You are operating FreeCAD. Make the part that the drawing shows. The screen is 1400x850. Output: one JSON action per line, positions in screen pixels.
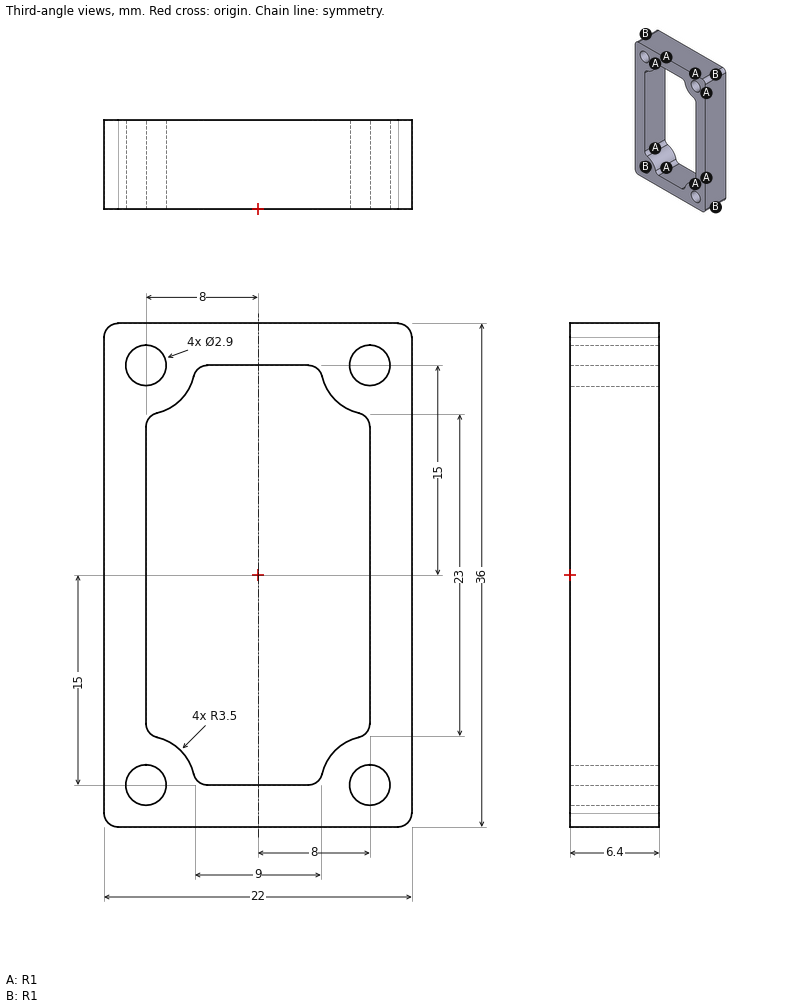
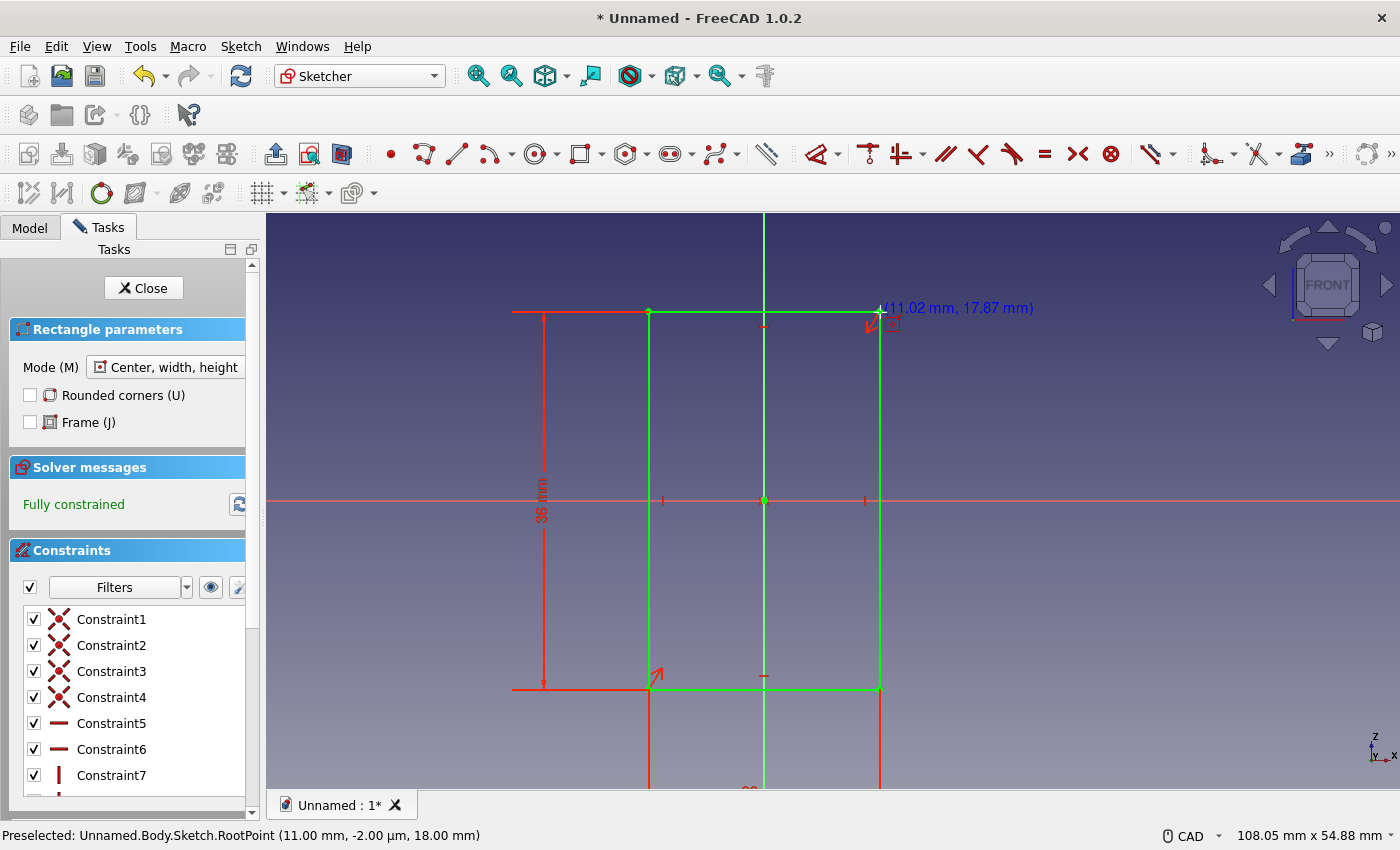
{"action": "left_click", "coordinate": [457, 154]}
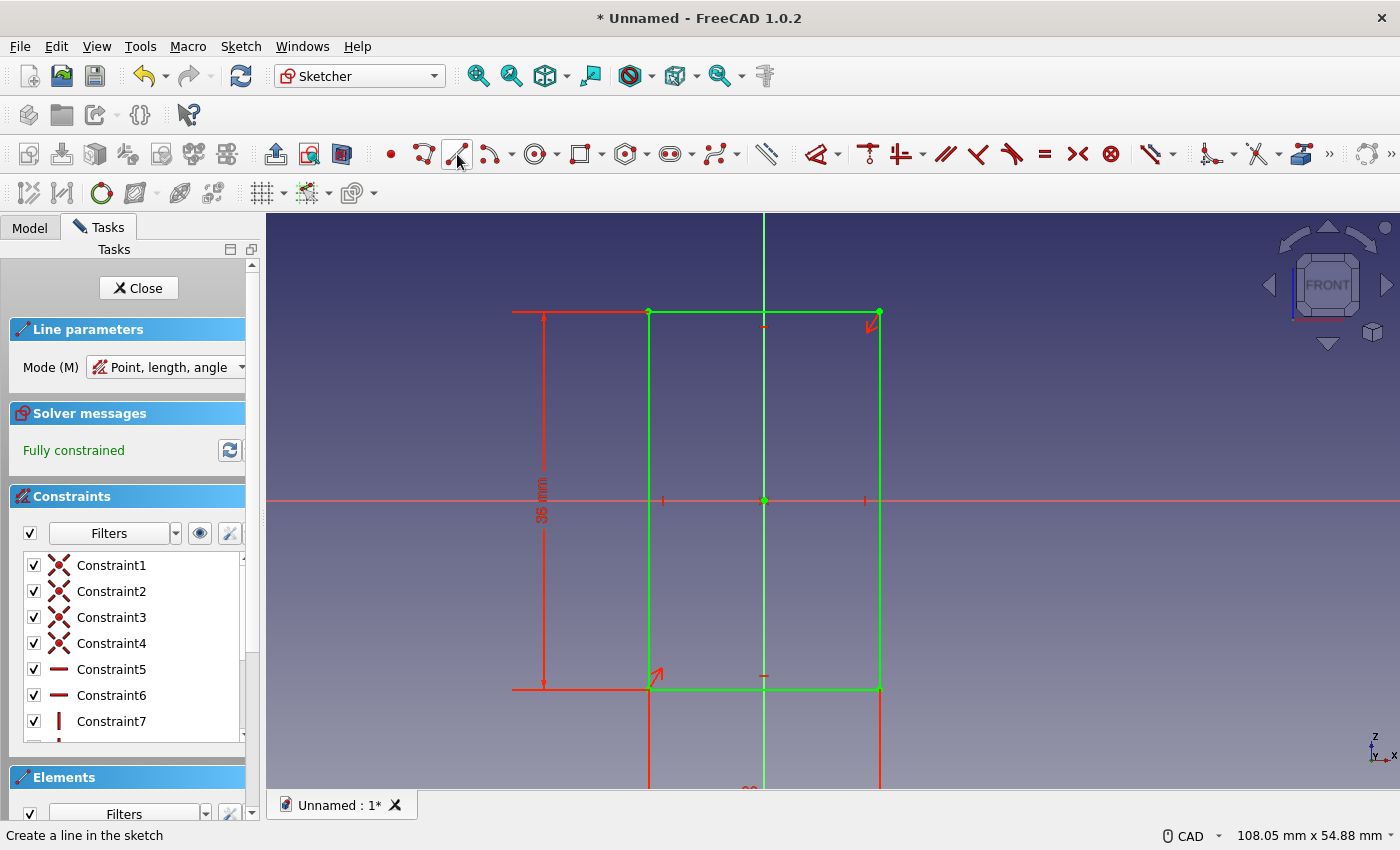
{"action": "left_click", "coordinate": [717, 658]}
{"action": "left_click", "coordinate": [812, 658]}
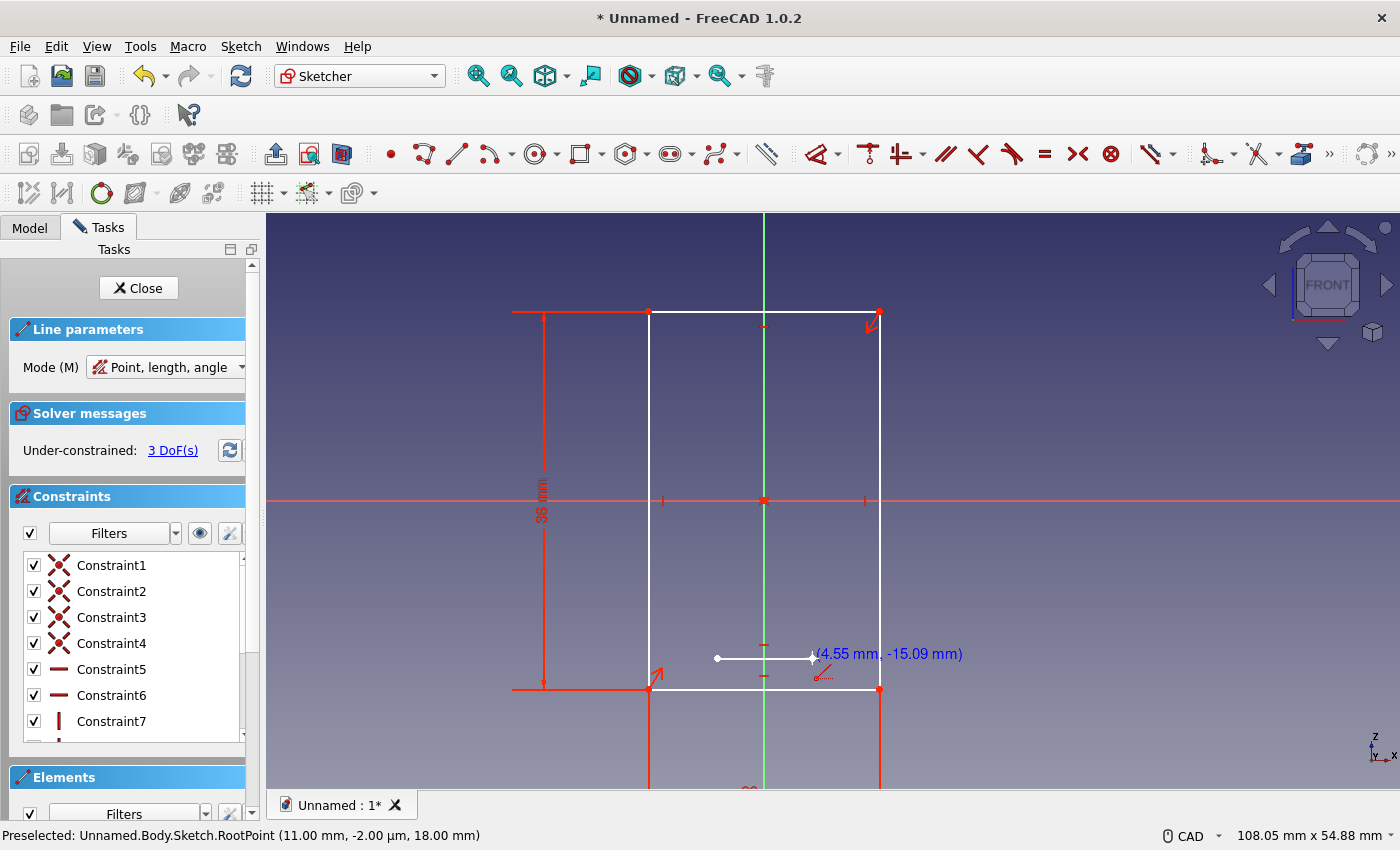
{"action": "left_click", "coordinate": [848, 621]}
{"action": "left_click", "coordinate": [848, 380]}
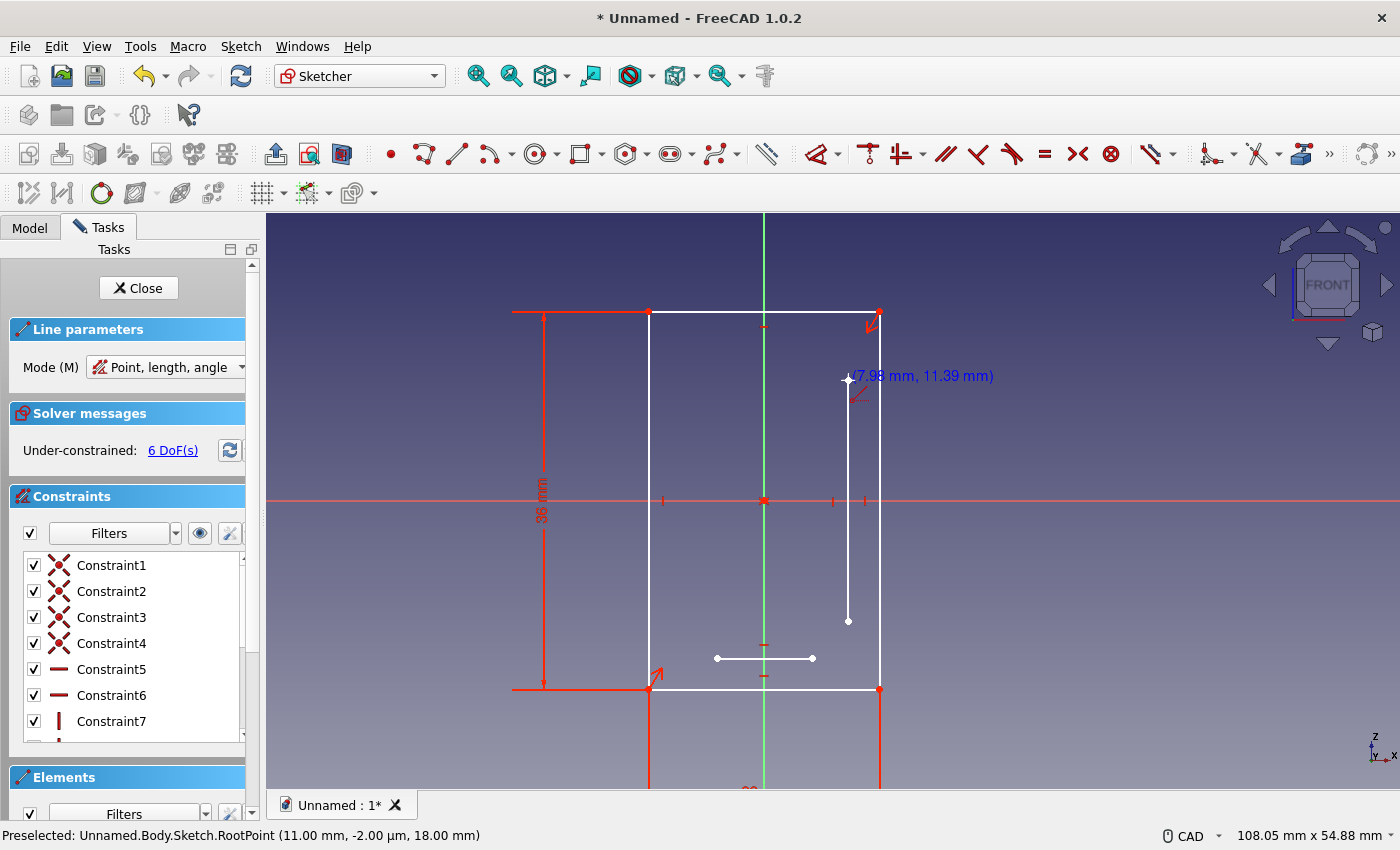
{"action": "left_click", "coordinate": [812, 343]}
{"action": "left_click", "coordinate": [717, 343]}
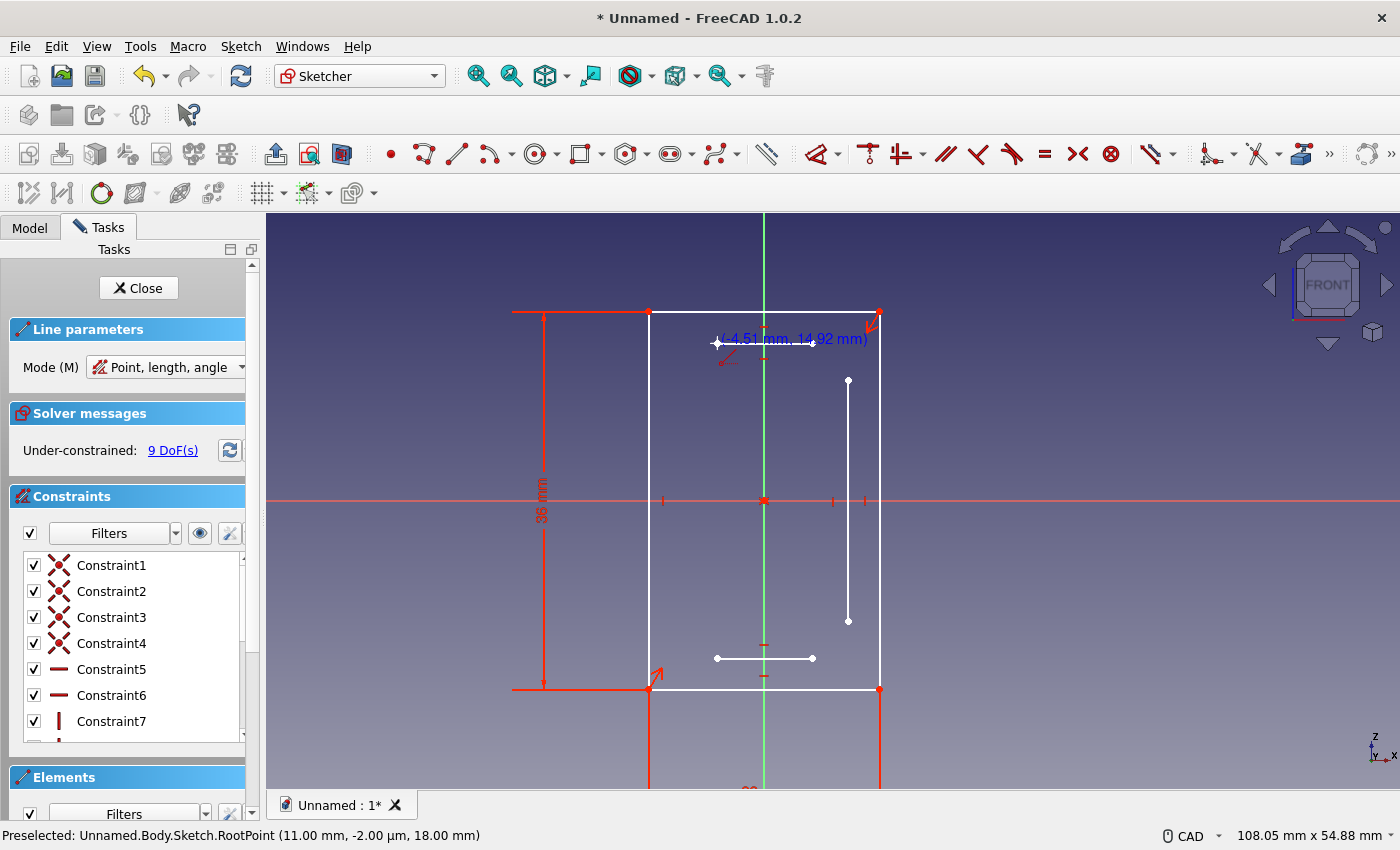
{"action": "left_click", "coordinate": [680, 380]}
{"action": "left_click", "coordinate": [680, 621]}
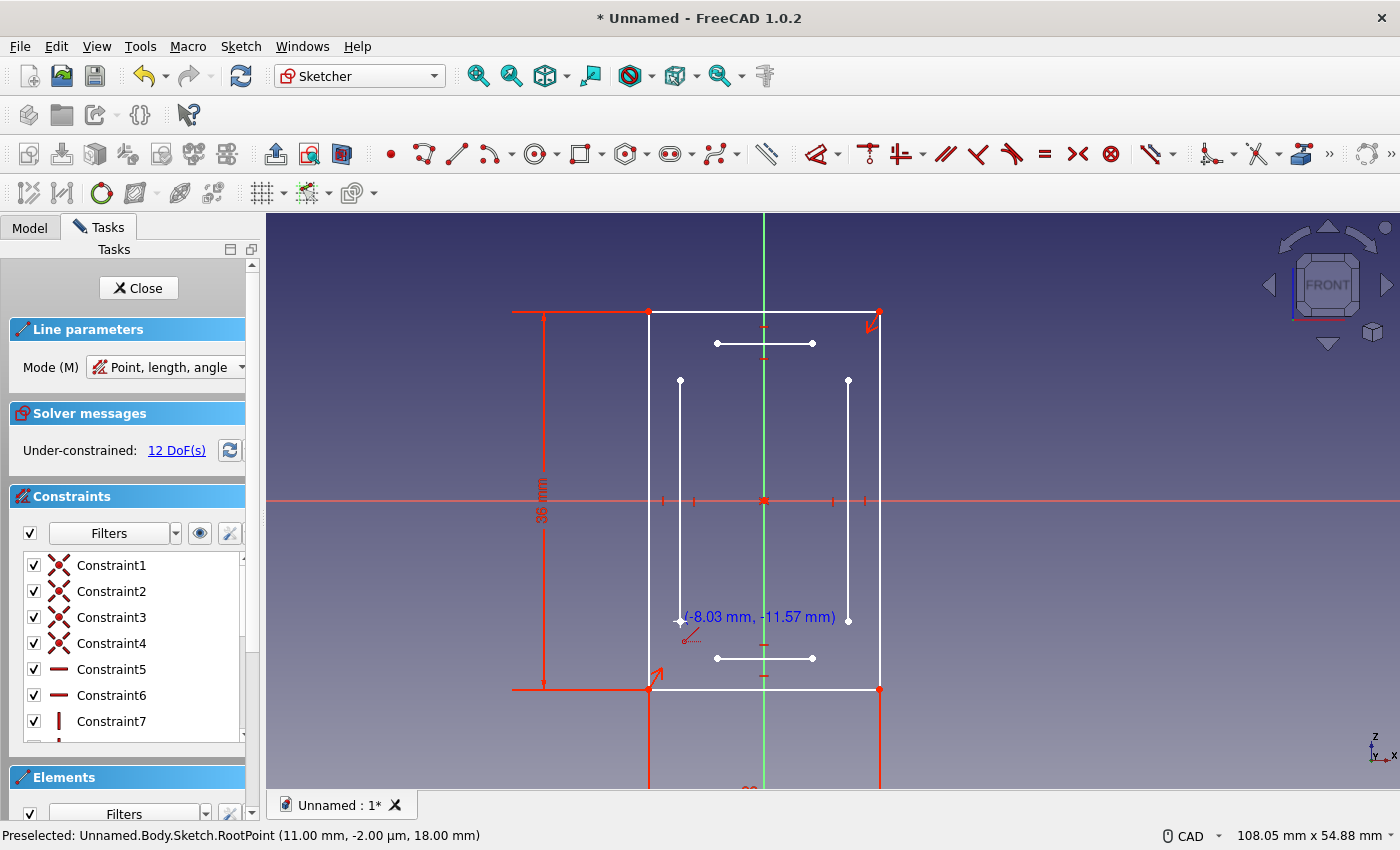
{"action": "key", "text": "g 3 a"}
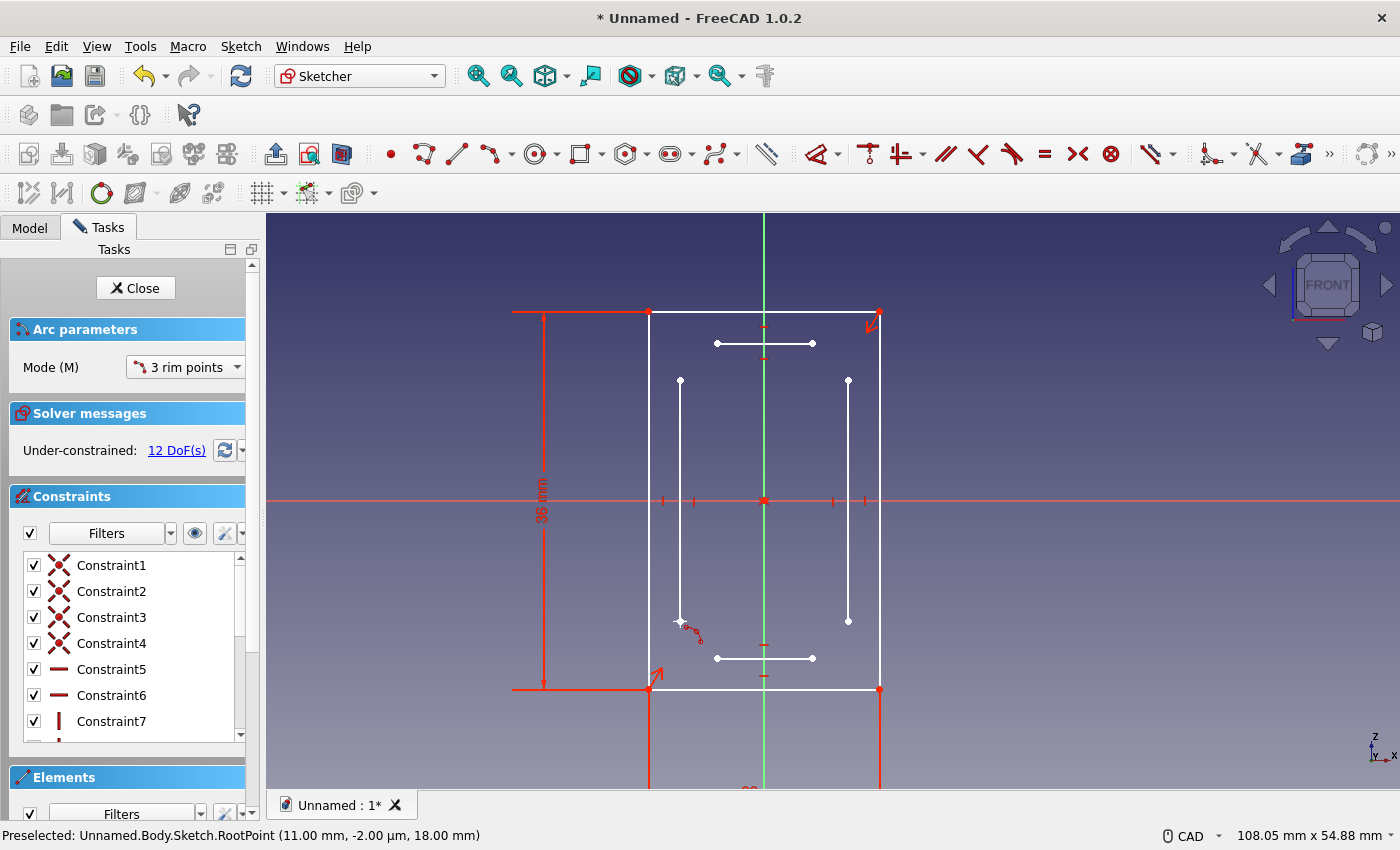
{"action": "left_click", "coordinate": [812, 659]}
{"action": "left_click", "coordinate": [848, 622]}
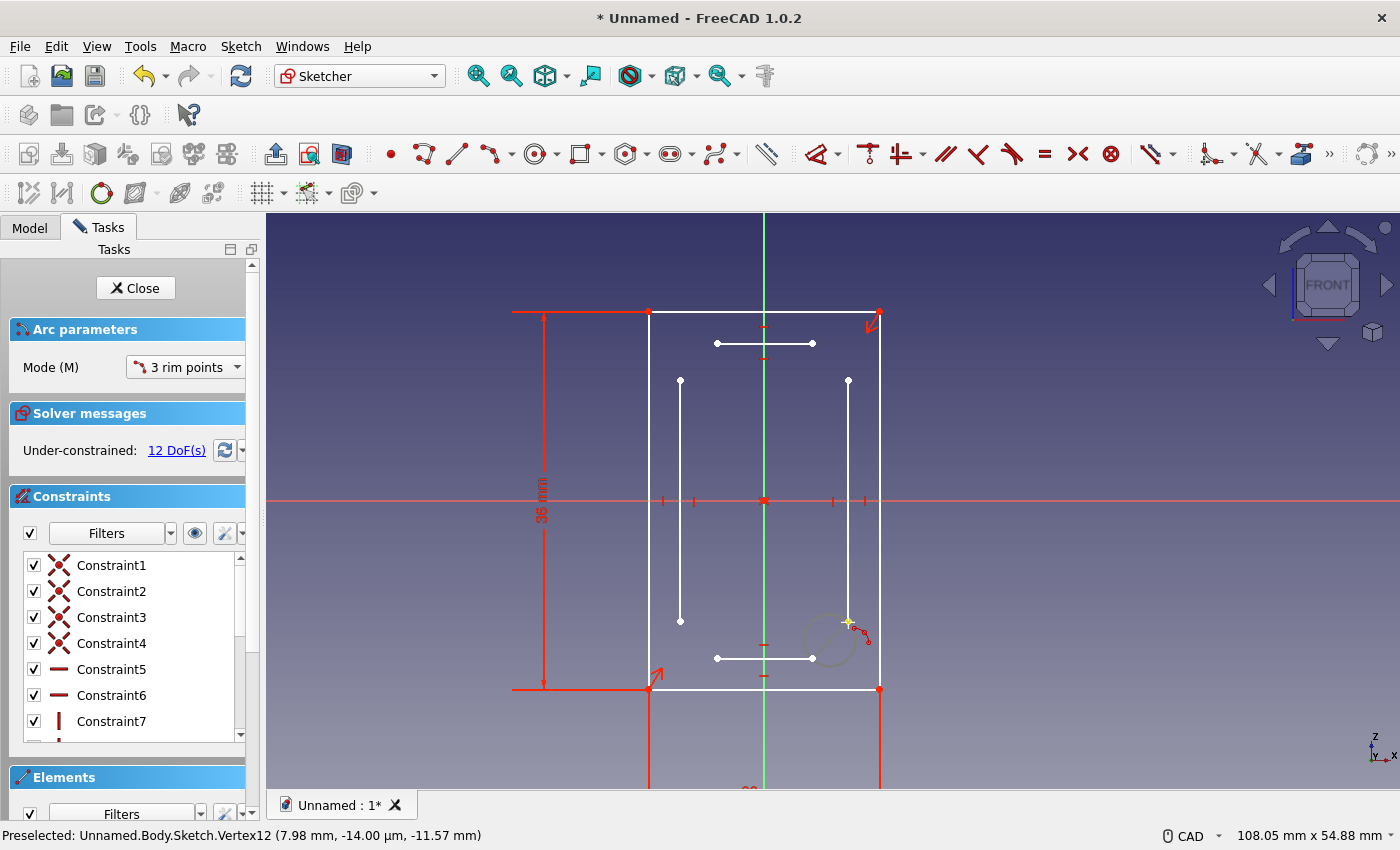
{"action": "scroll", "coordinate": [822, 632], "scroll_direction": "up", "scroll_amount": 2}